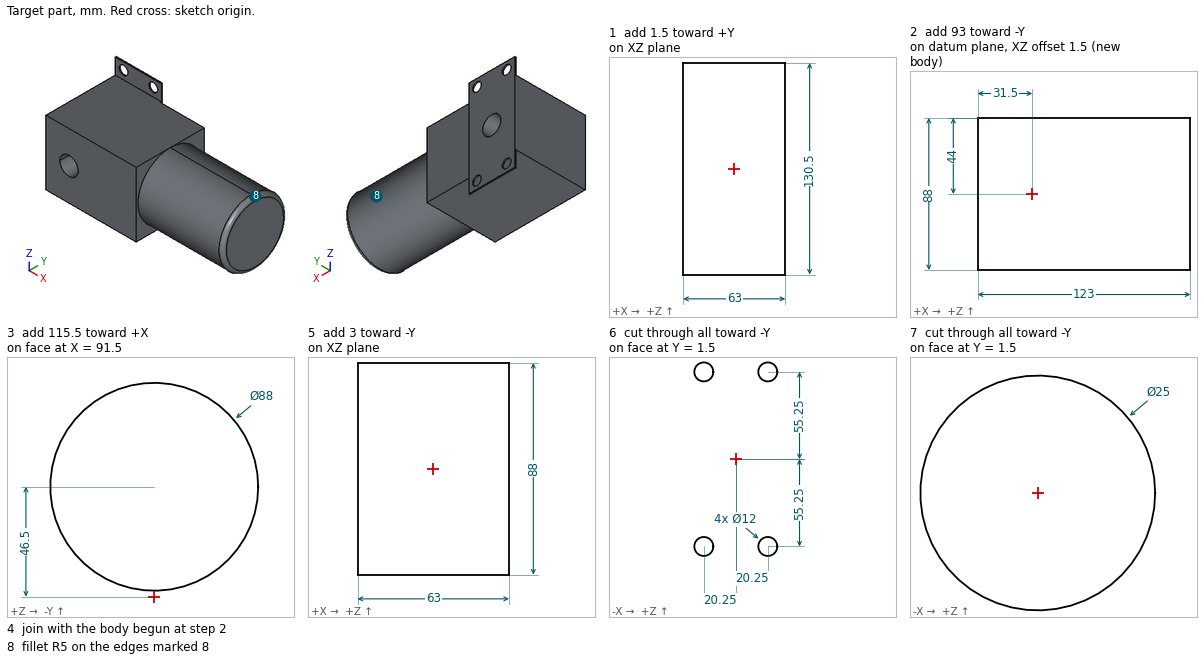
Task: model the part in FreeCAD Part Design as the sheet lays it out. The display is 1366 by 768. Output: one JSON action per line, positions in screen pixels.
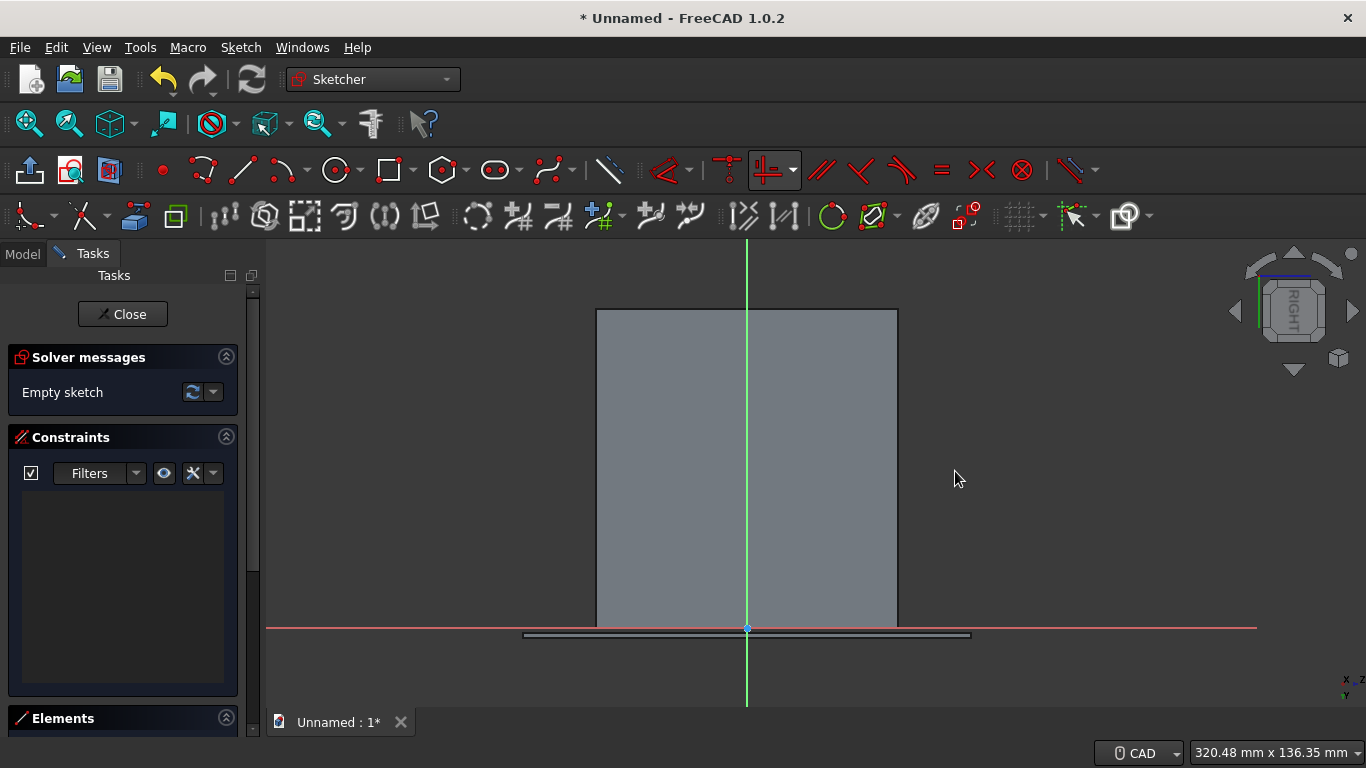
{"action": "left_click", "coordinate": [336, 170]}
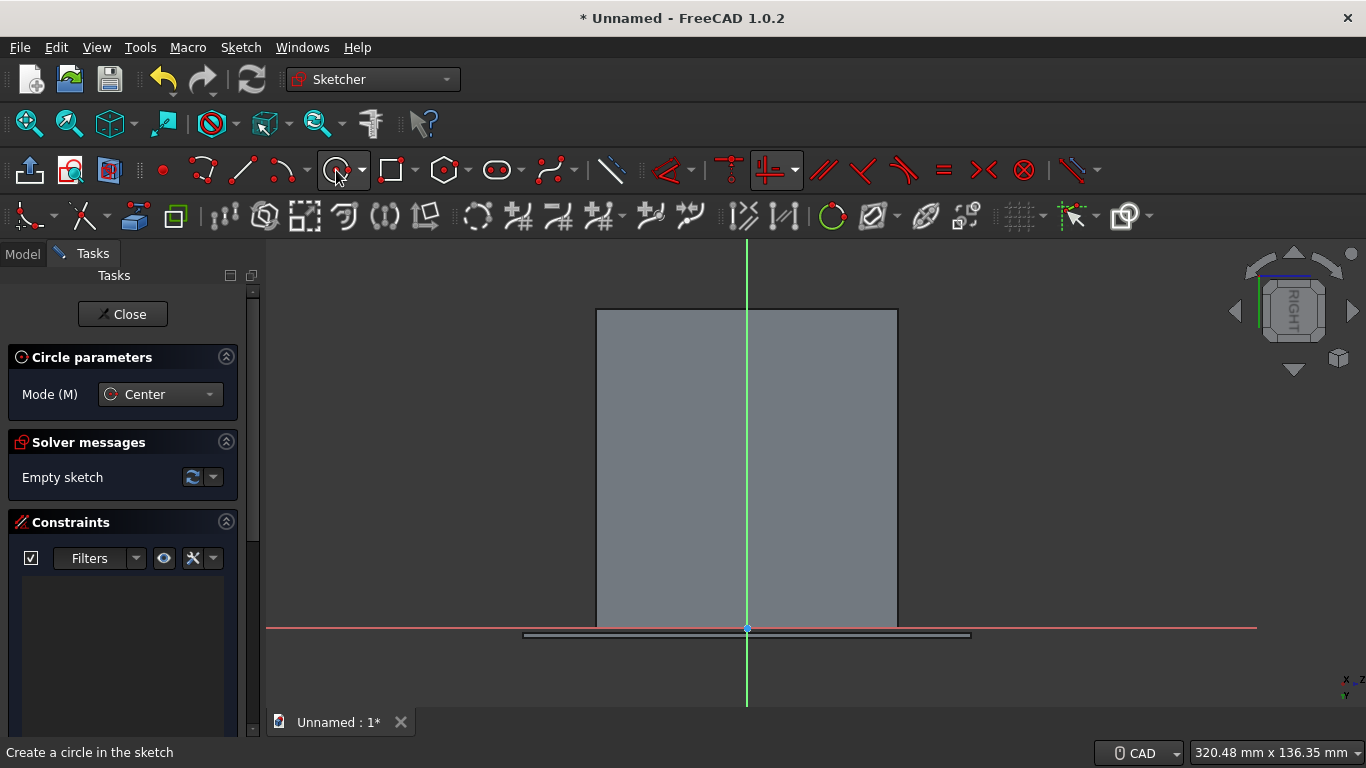
{"action": "left_click", "coordinate": [747, 469]}
{"action": "left_click", "coordinate": [854, 362]}
{"action": "key", "text": "Escape"}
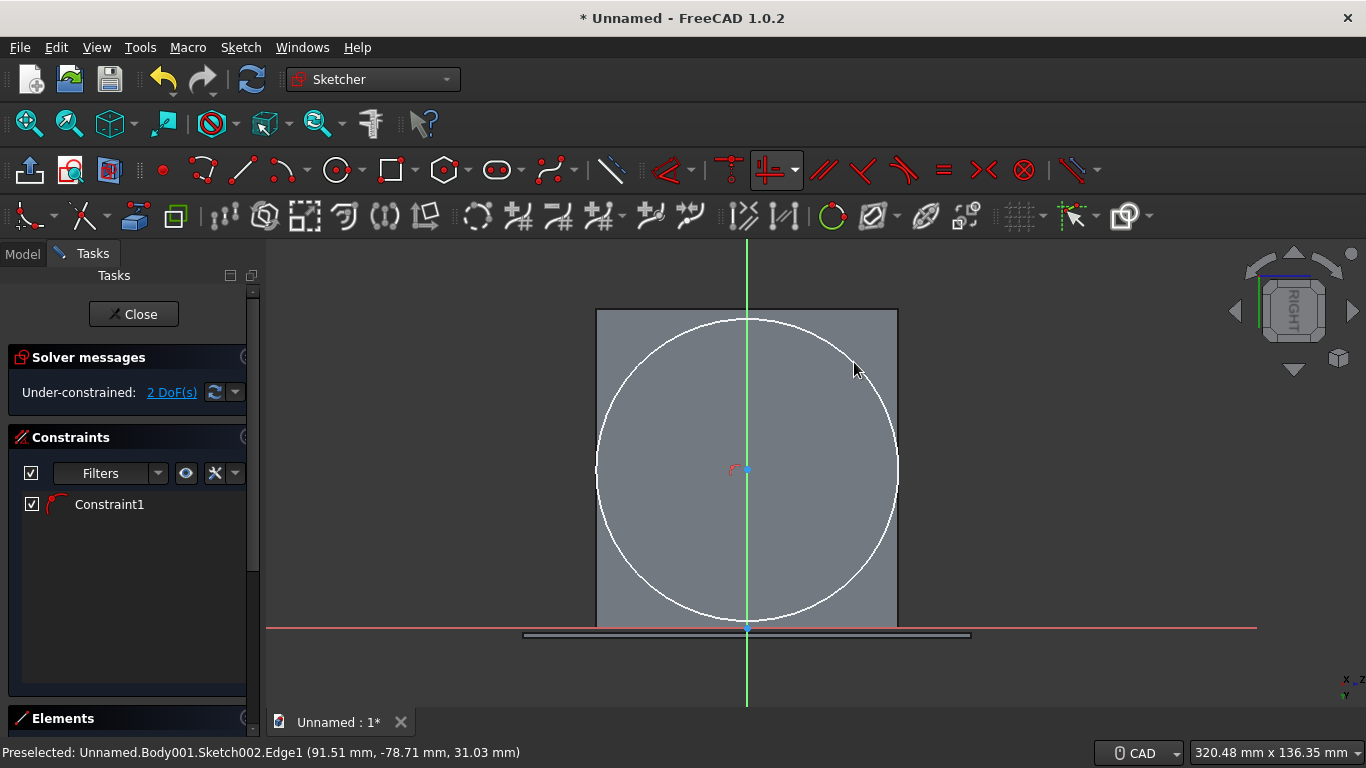
{"action": "left_click", "coordinate": [666, 170]}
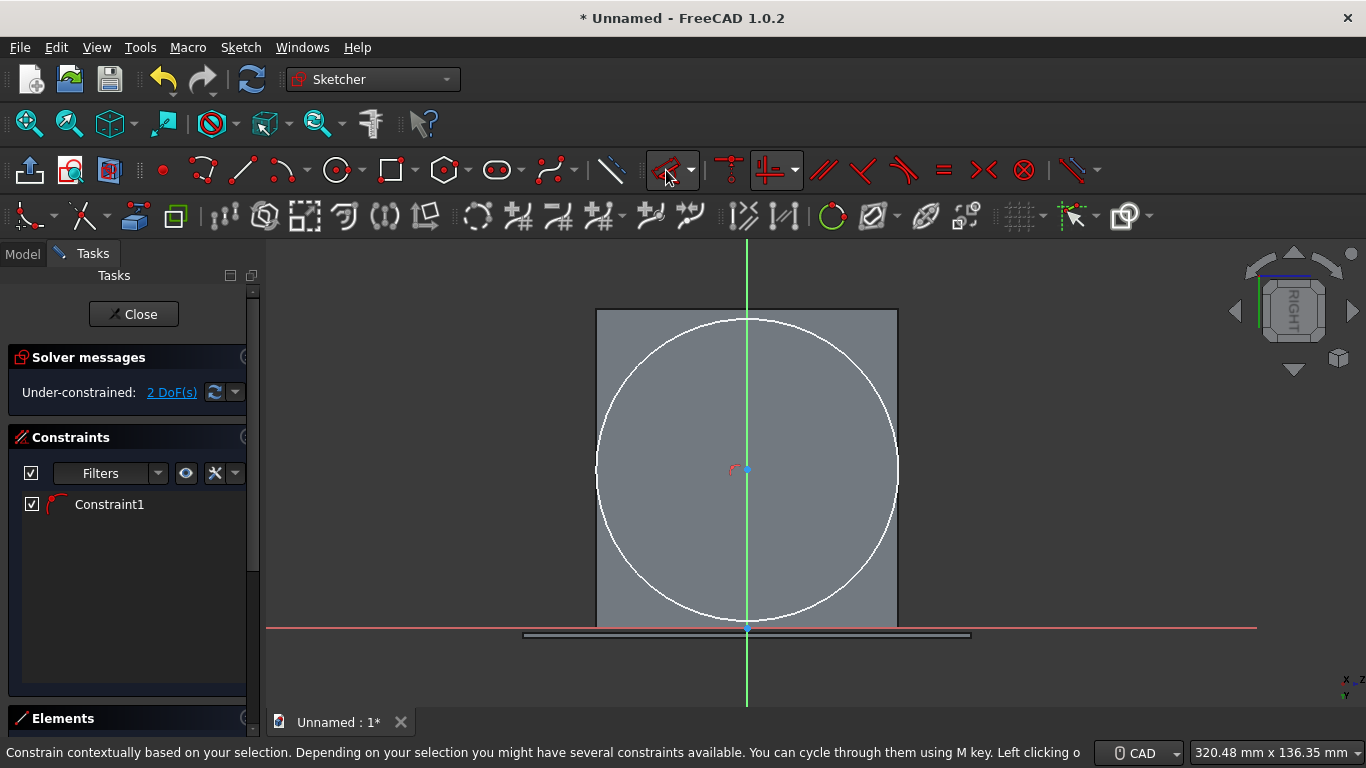
{"action": "left_click", "coordinate": [854, 363]}
{"action": "left_click", "coordinate": [877, 340]}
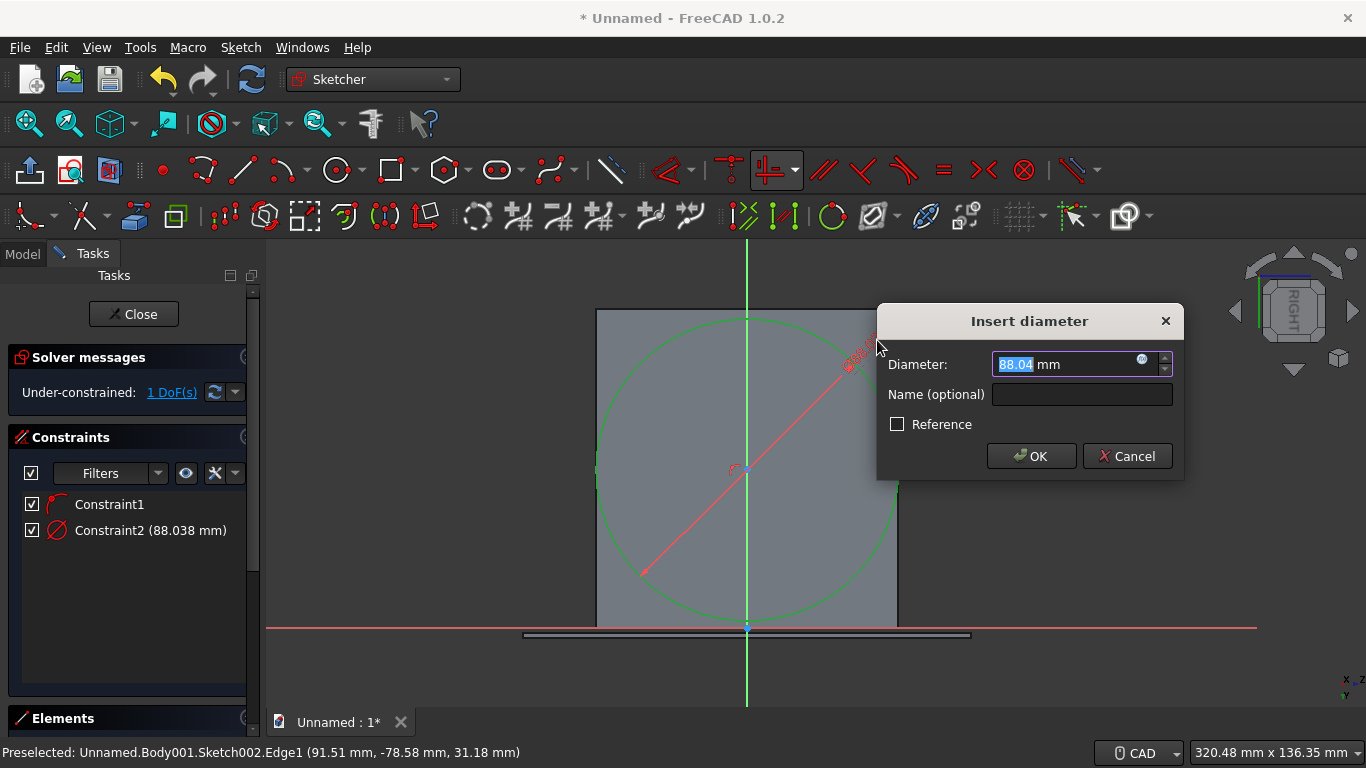
{"action": "type", "text": "88"}
{"action": "key", "text": "Return"}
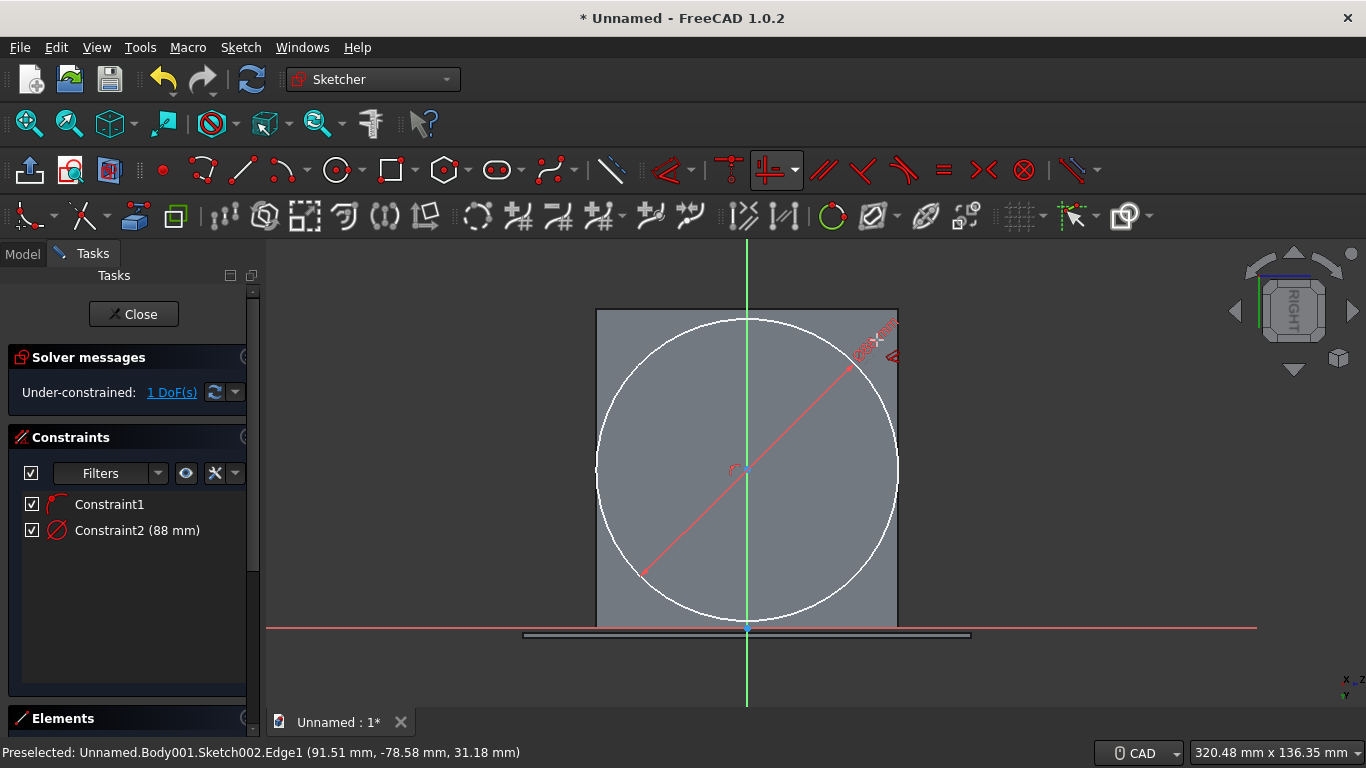
{"action": "left_click", "coordinate": [747, 470]}
{"action": "left_click", "coordinate": [781, 549]}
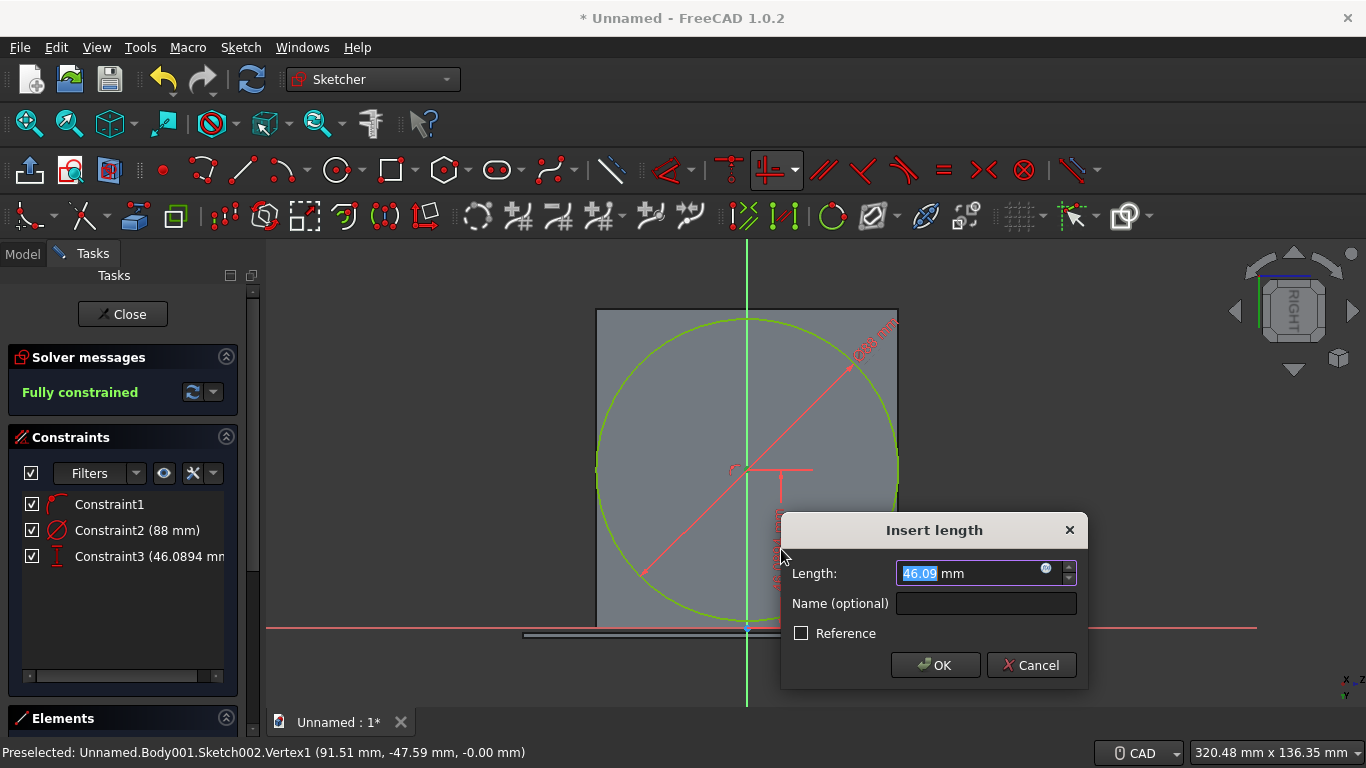
{"action": "type", "text": "46.5"}
{"action": "key", "text": "Return"}
{"action": "key", "text": "Escape"}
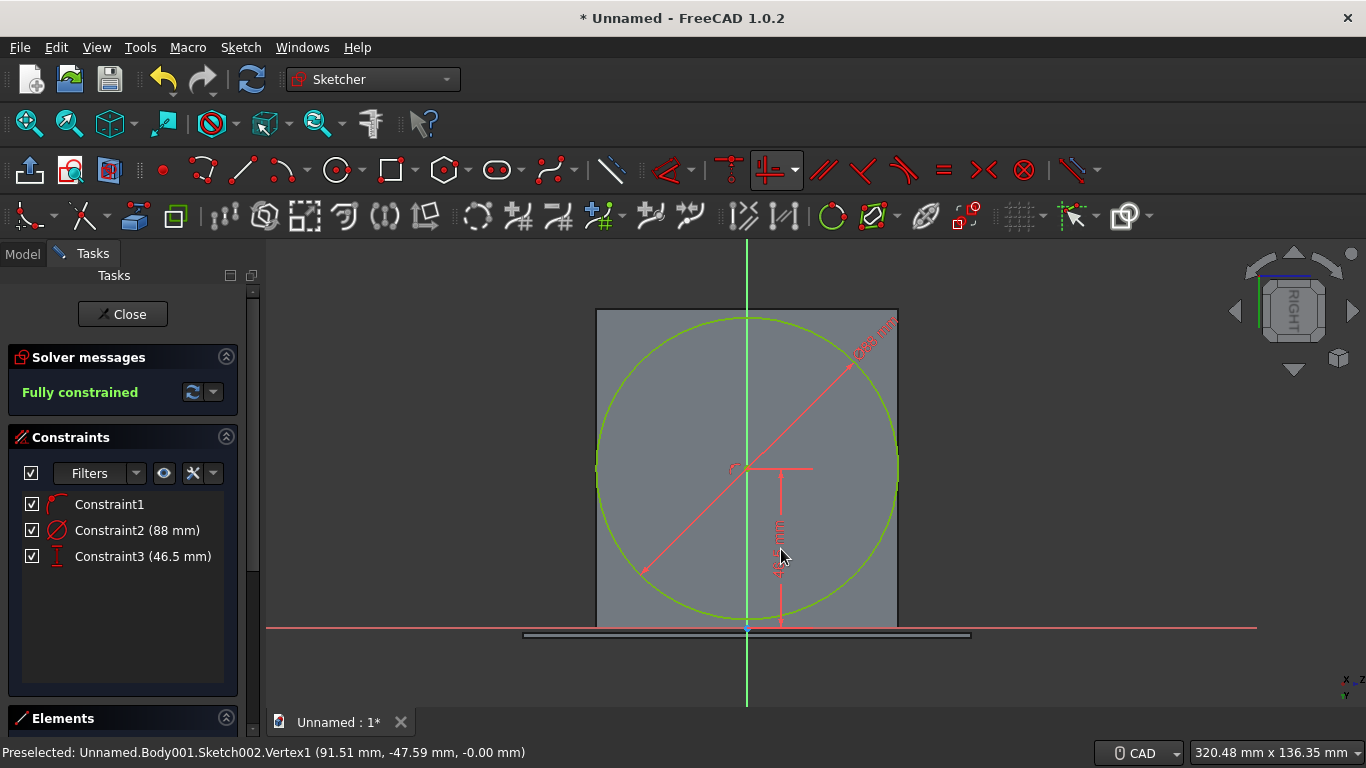
{"action": "left_click", "coordinate": [123, 314]}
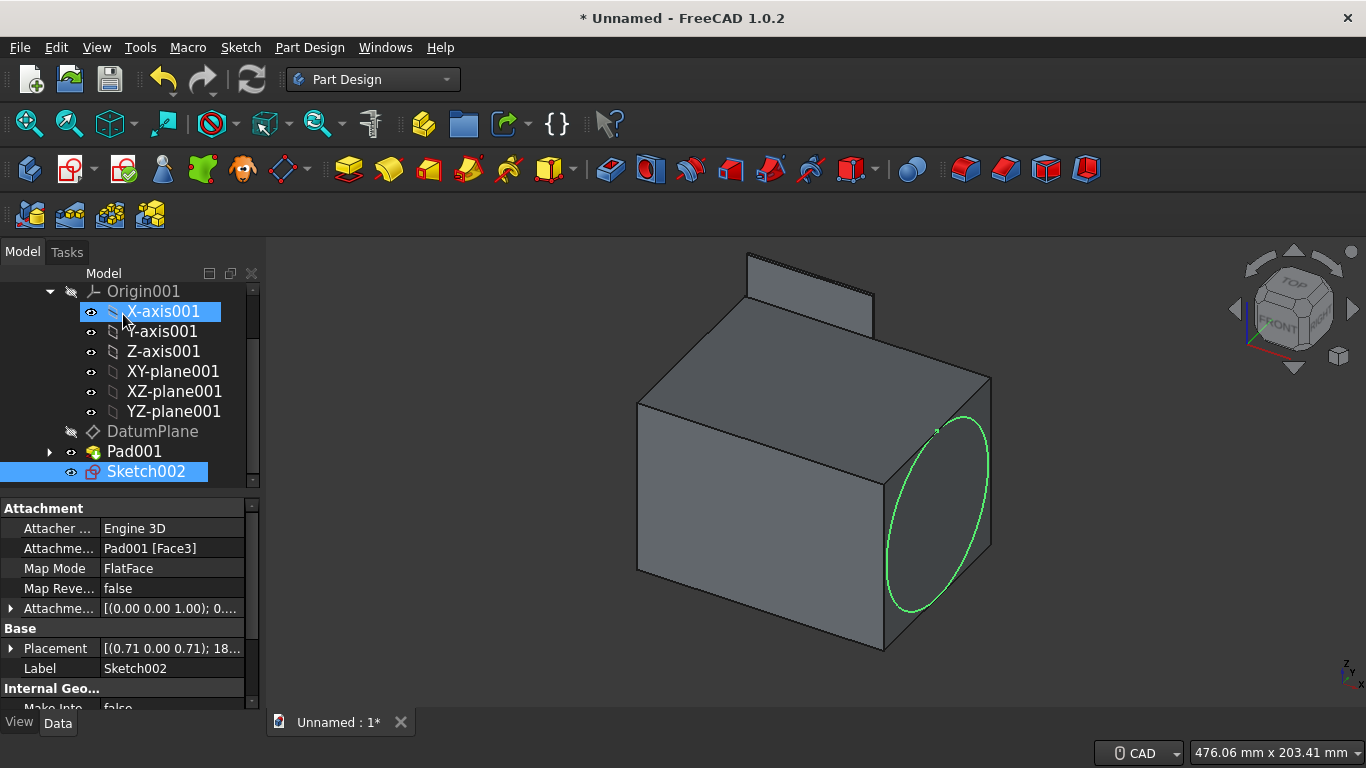
{"action": "left_click", "coordinate": [350, 170]}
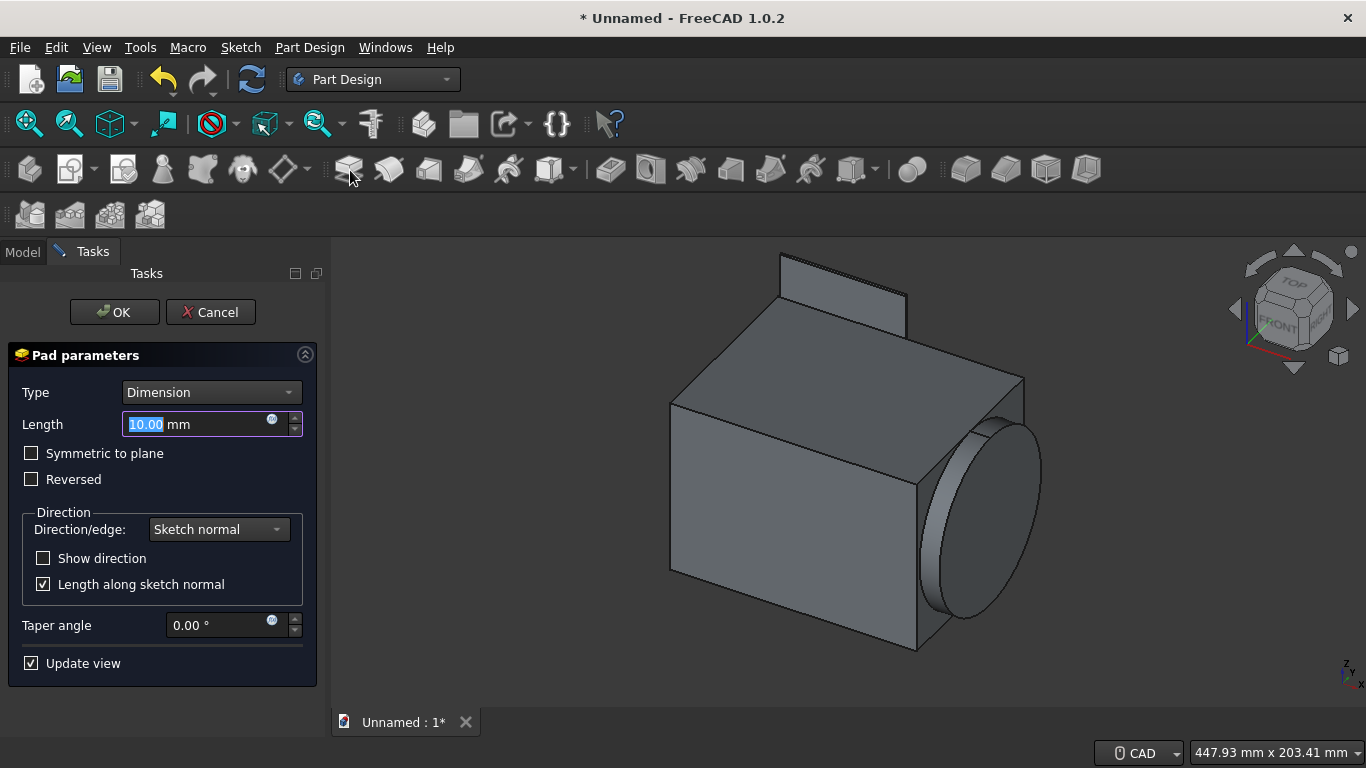
{"action": "type", "text": "115.5"}
{"action": "key", "text": "Tab"}